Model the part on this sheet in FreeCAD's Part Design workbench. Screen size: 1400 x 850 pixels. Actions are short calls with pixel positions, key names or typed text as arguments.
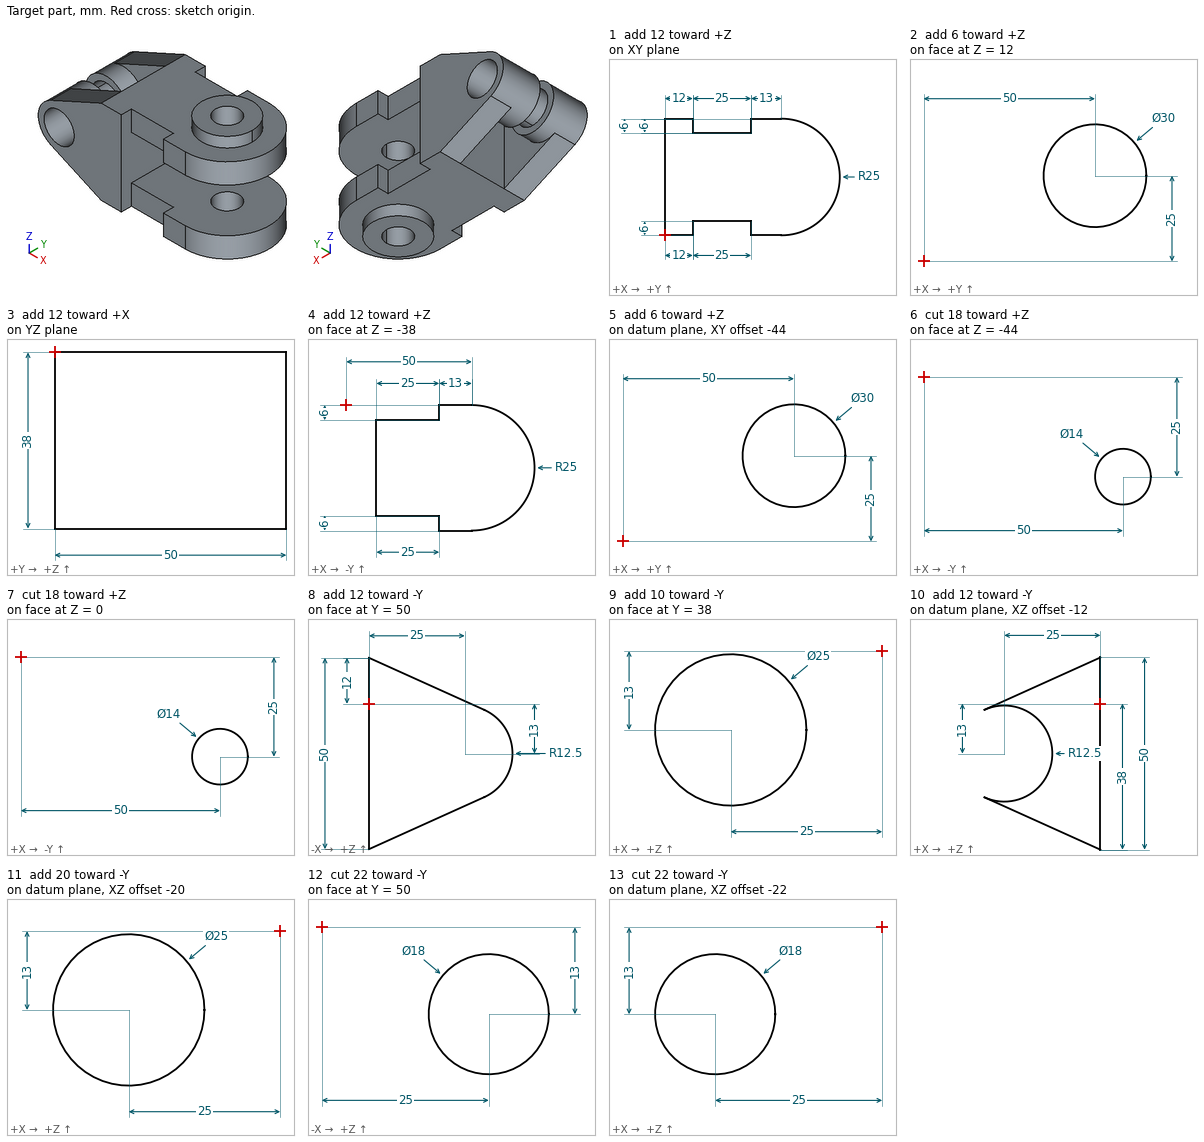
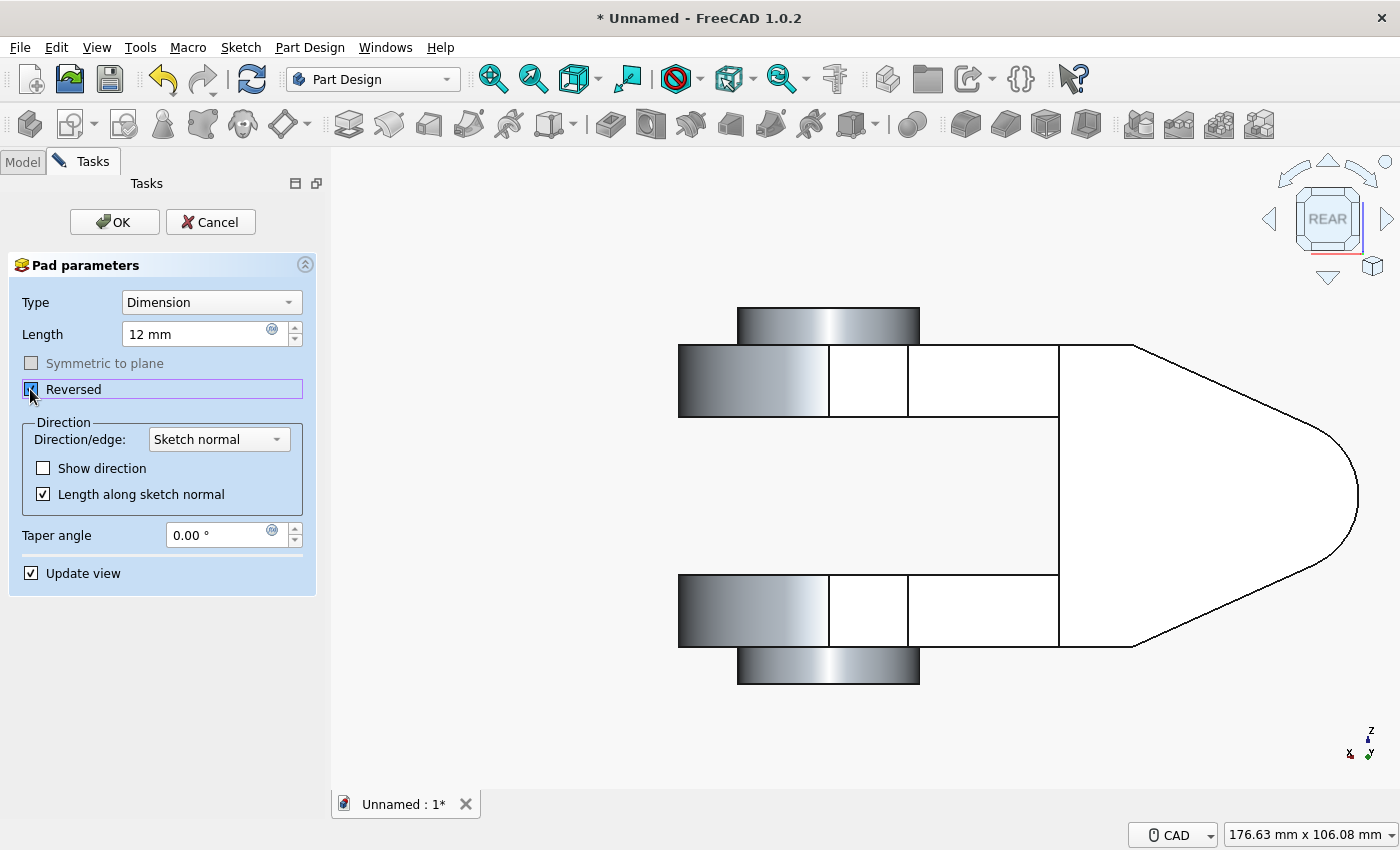
click(115, 222)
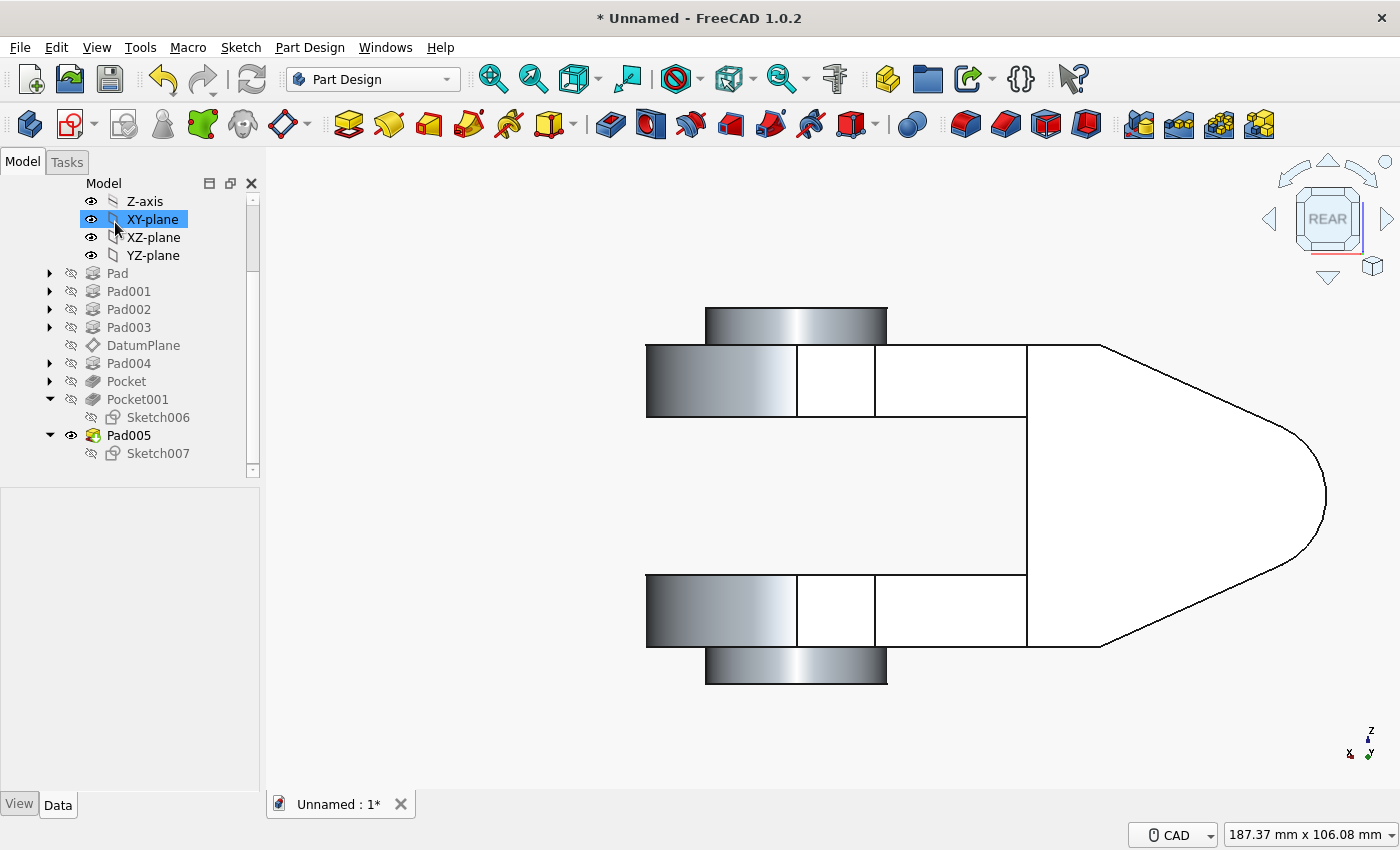
key(0)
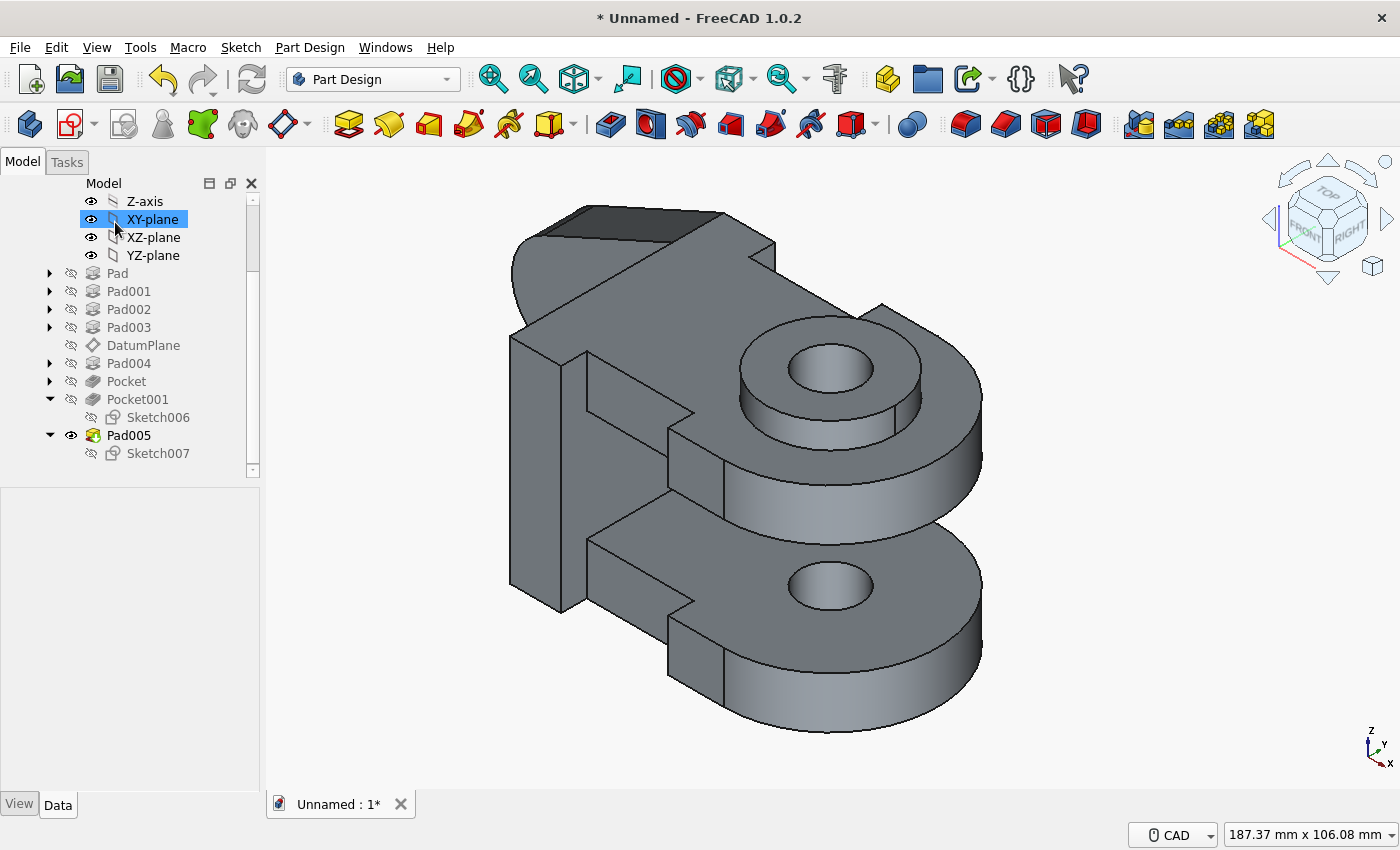
key(v)
key(f)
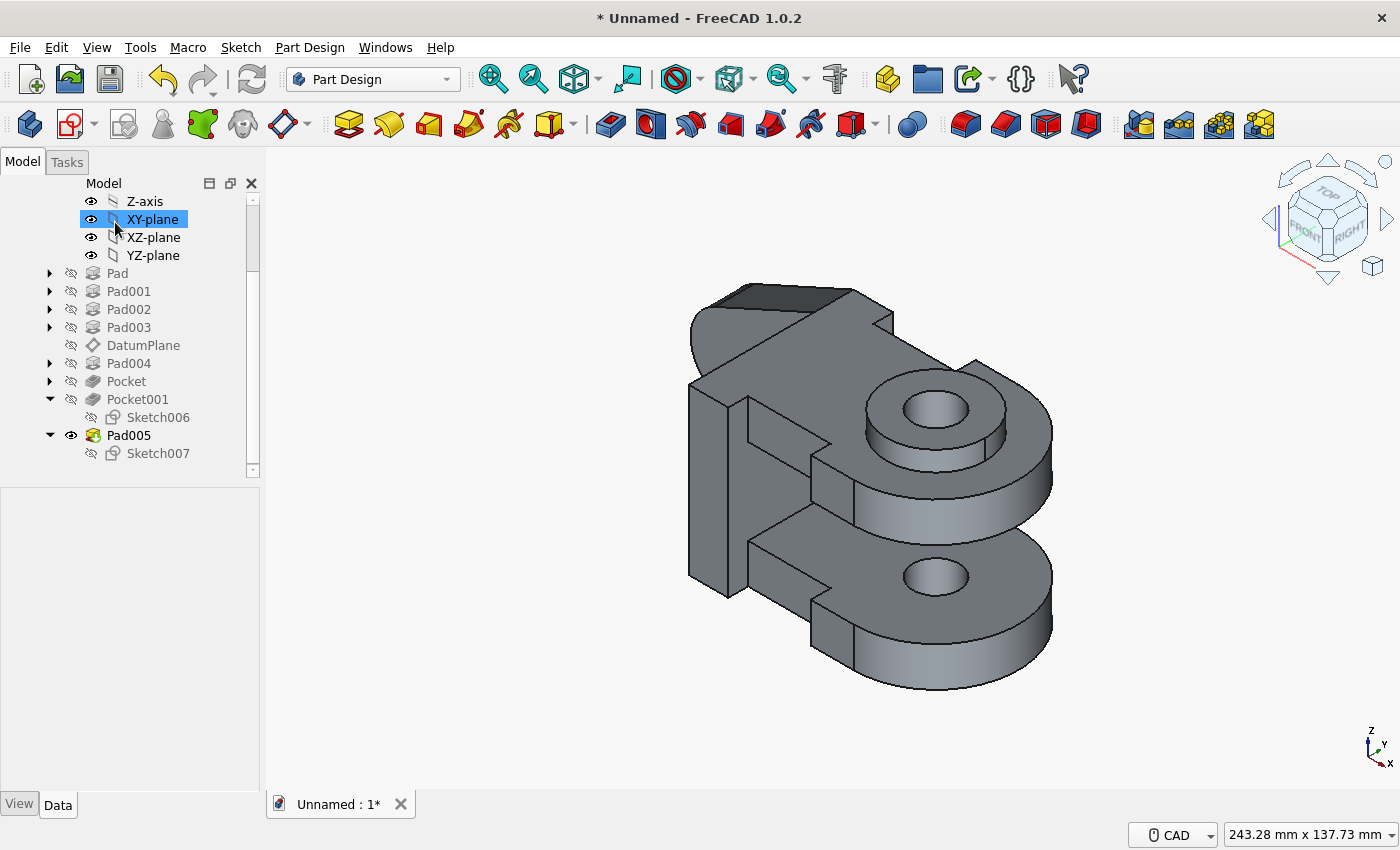
key(1)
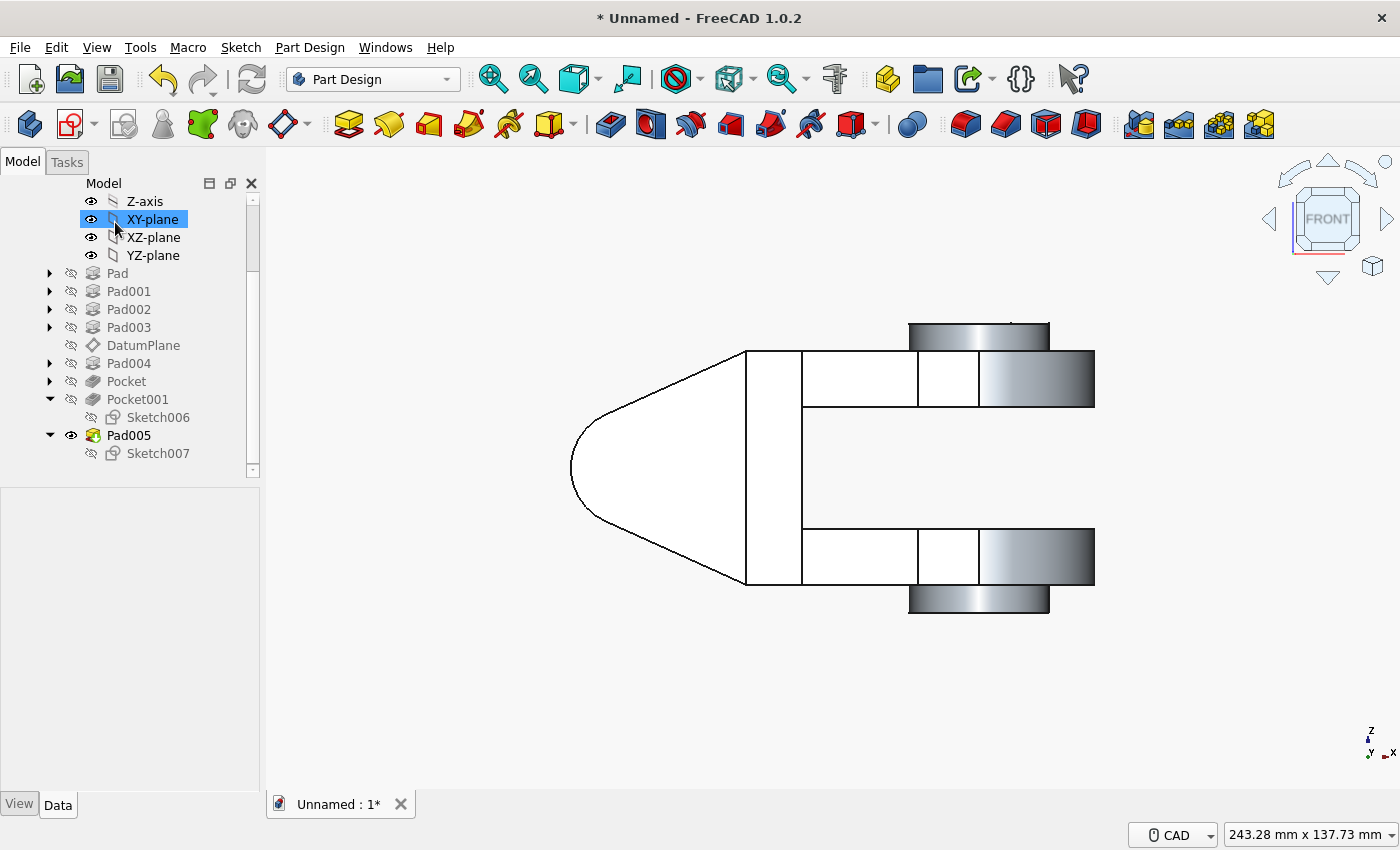
click(658, 467)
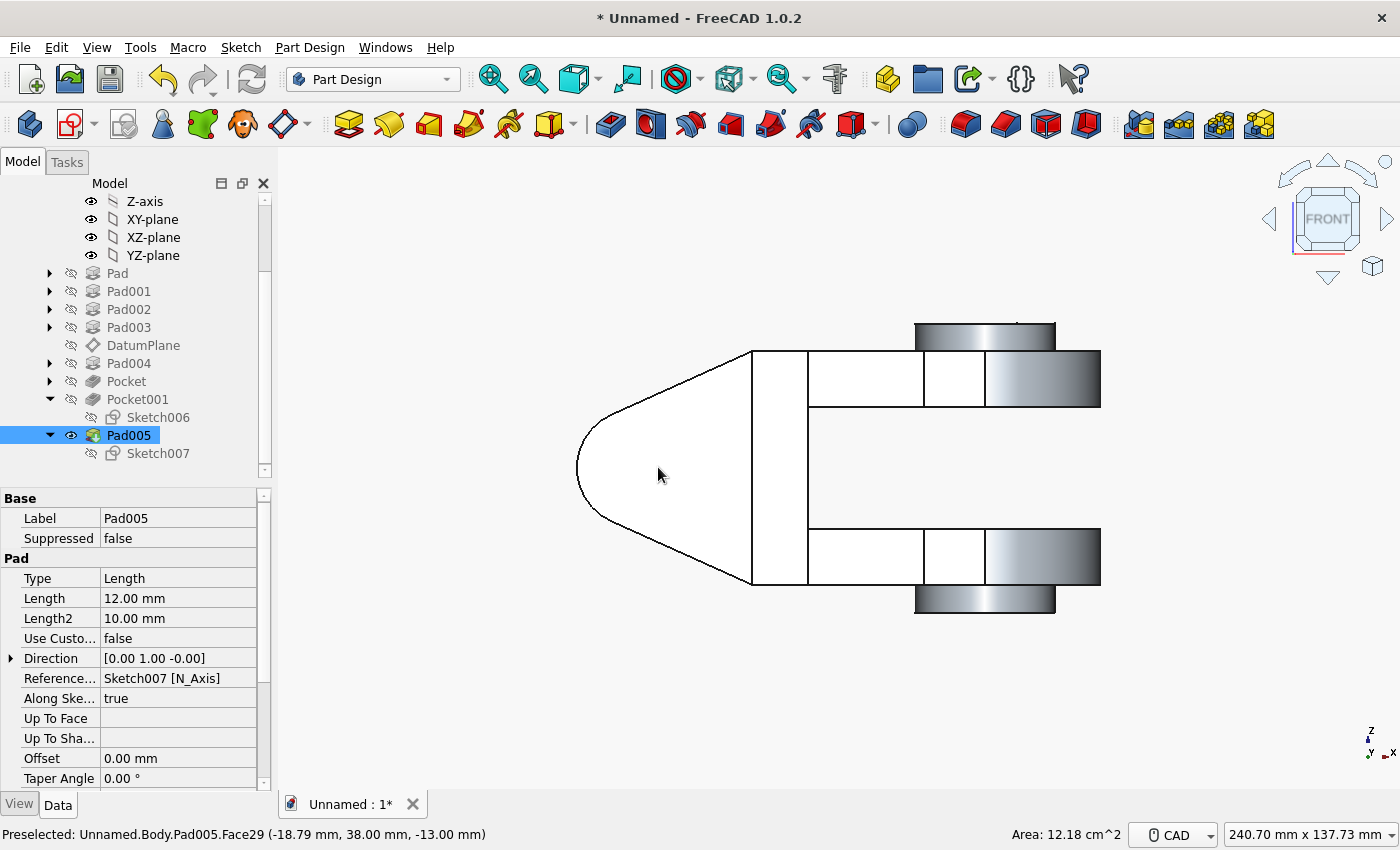
click(70, 124)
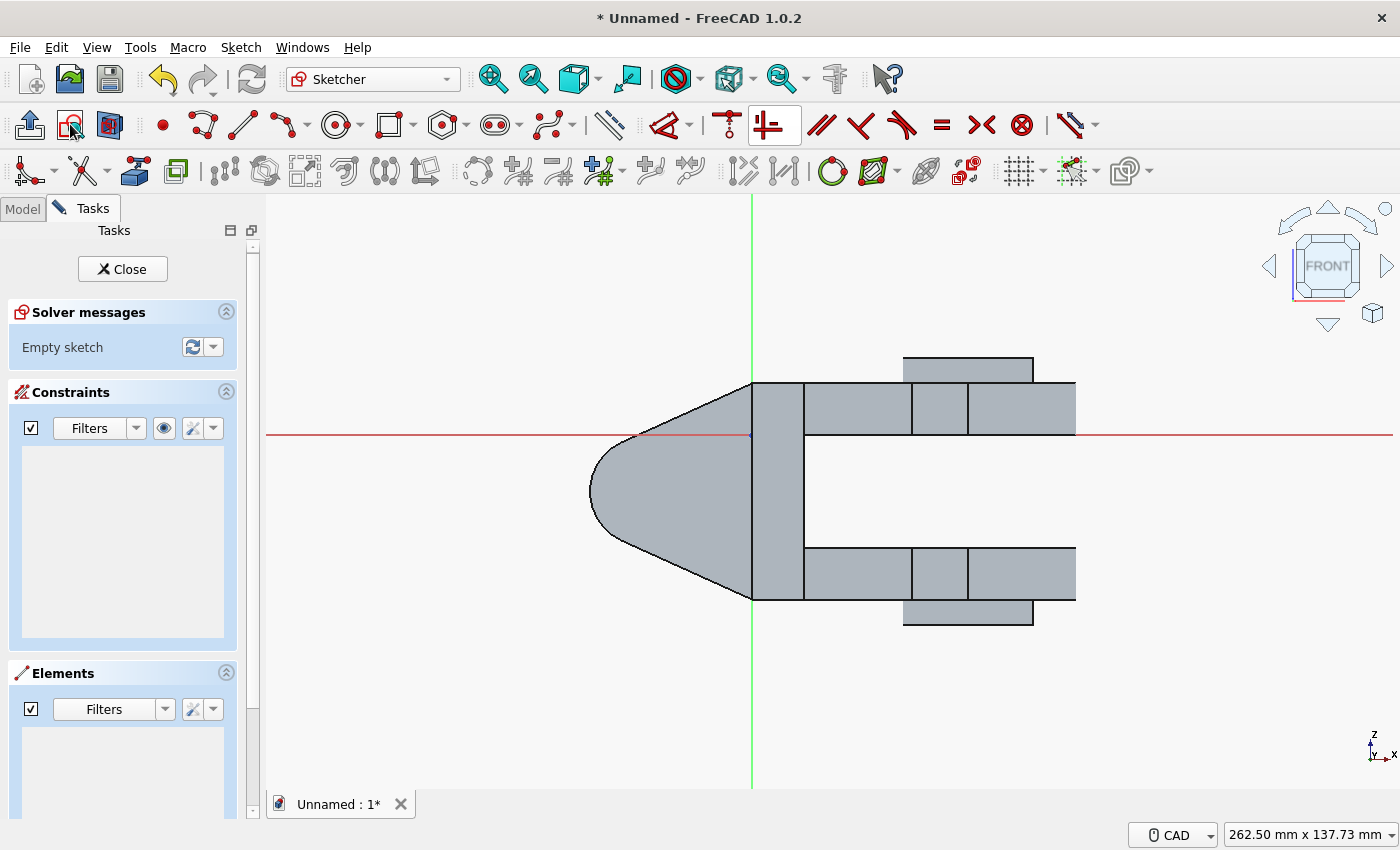
click(110, 126)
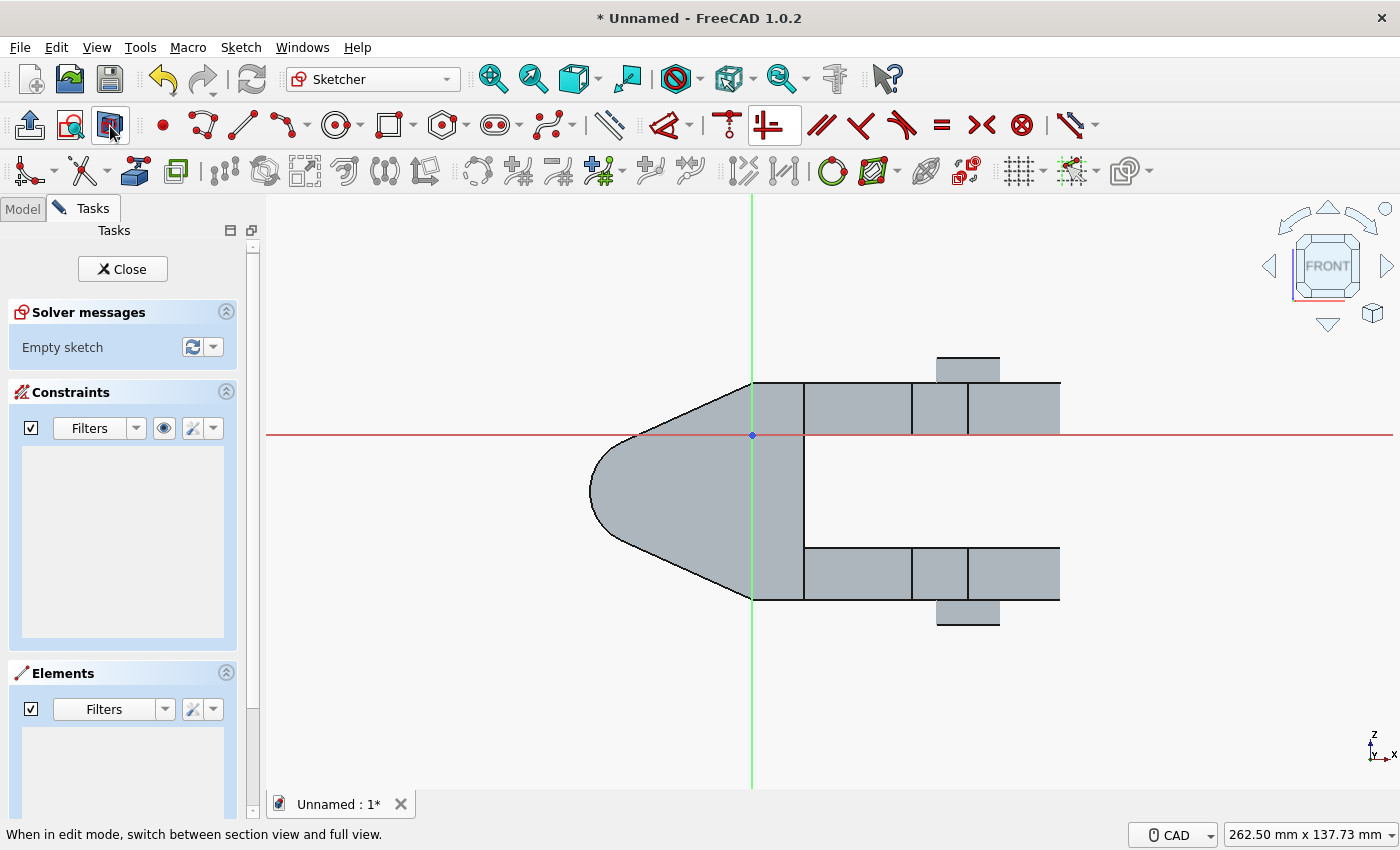
scroll(631, 490, up, 6)